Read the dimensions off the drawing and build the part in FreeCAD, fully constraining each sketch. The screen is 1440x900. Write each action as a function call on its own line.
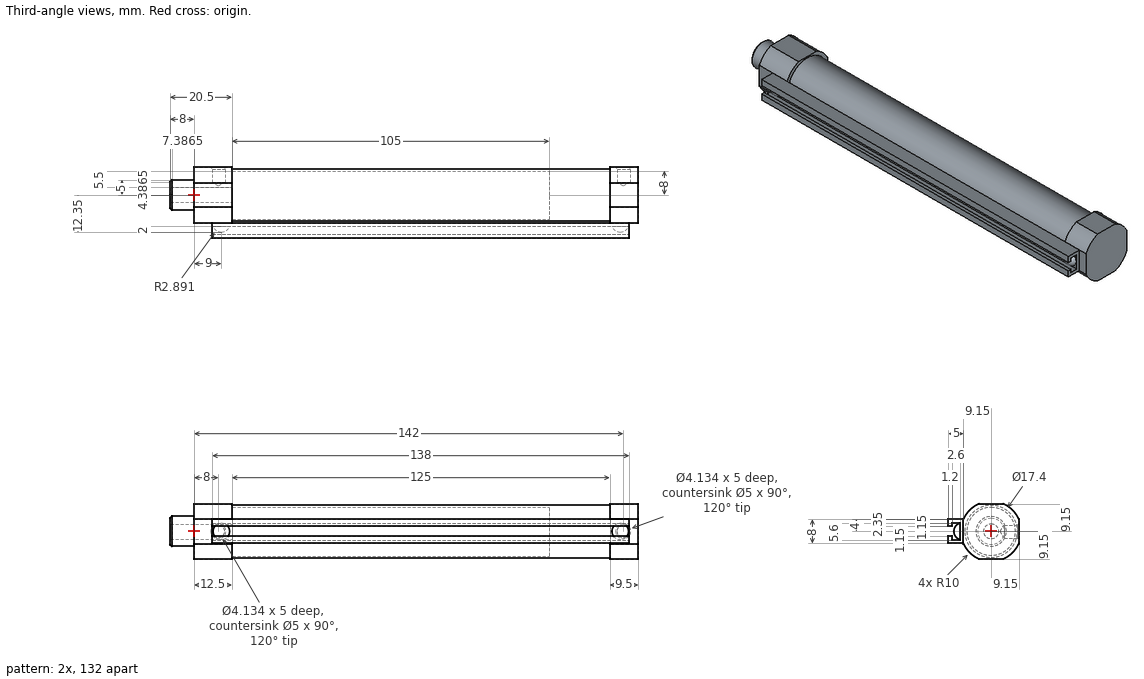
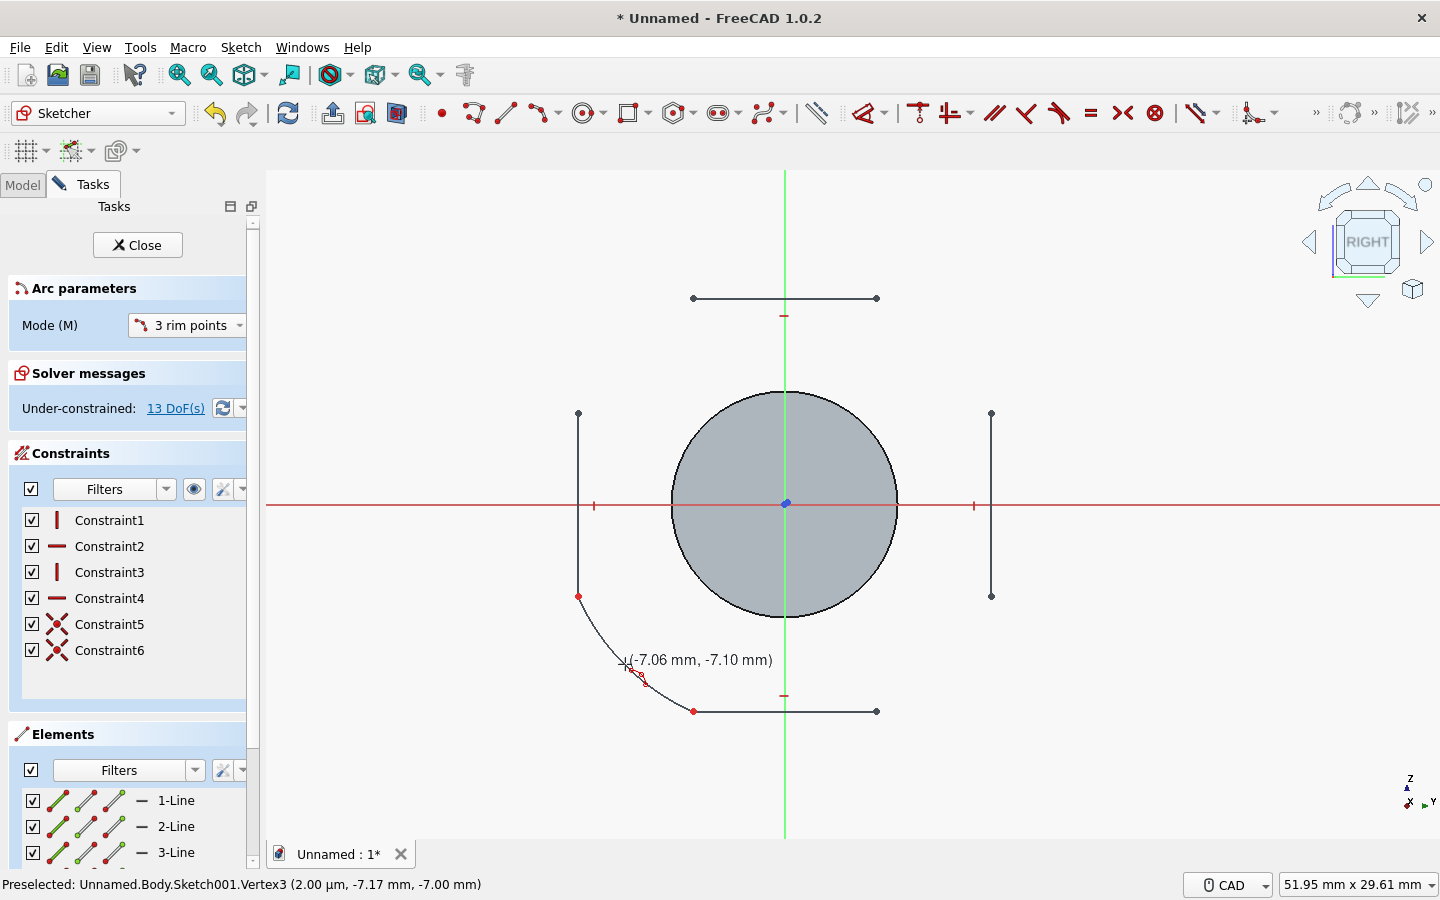
click(876, 712)
click(991, 597)
click(944, 664)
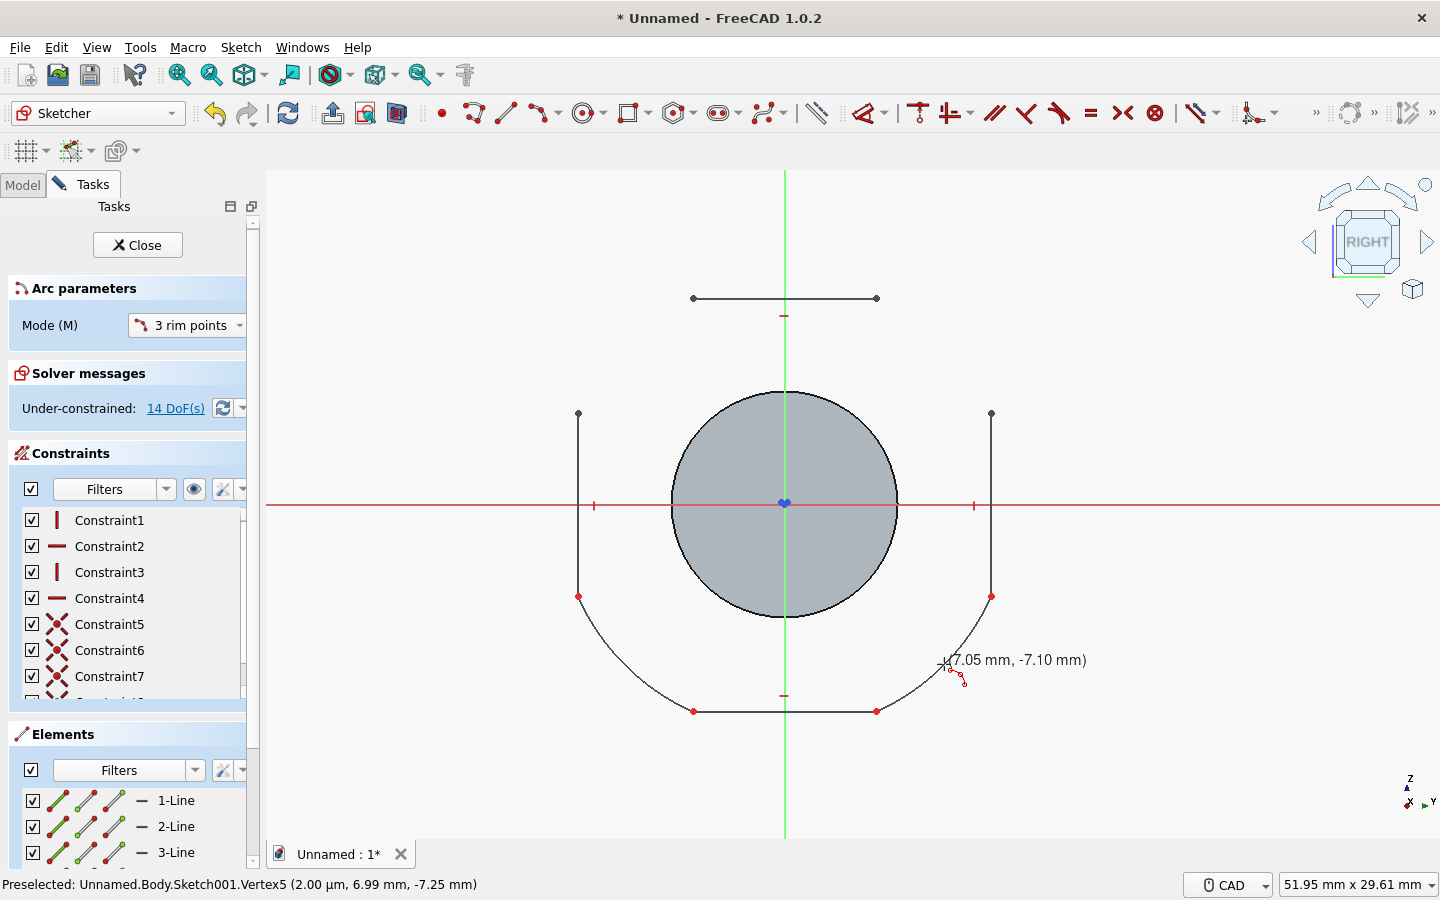
click(991, 414)
click(876, 299)
click(944, 345)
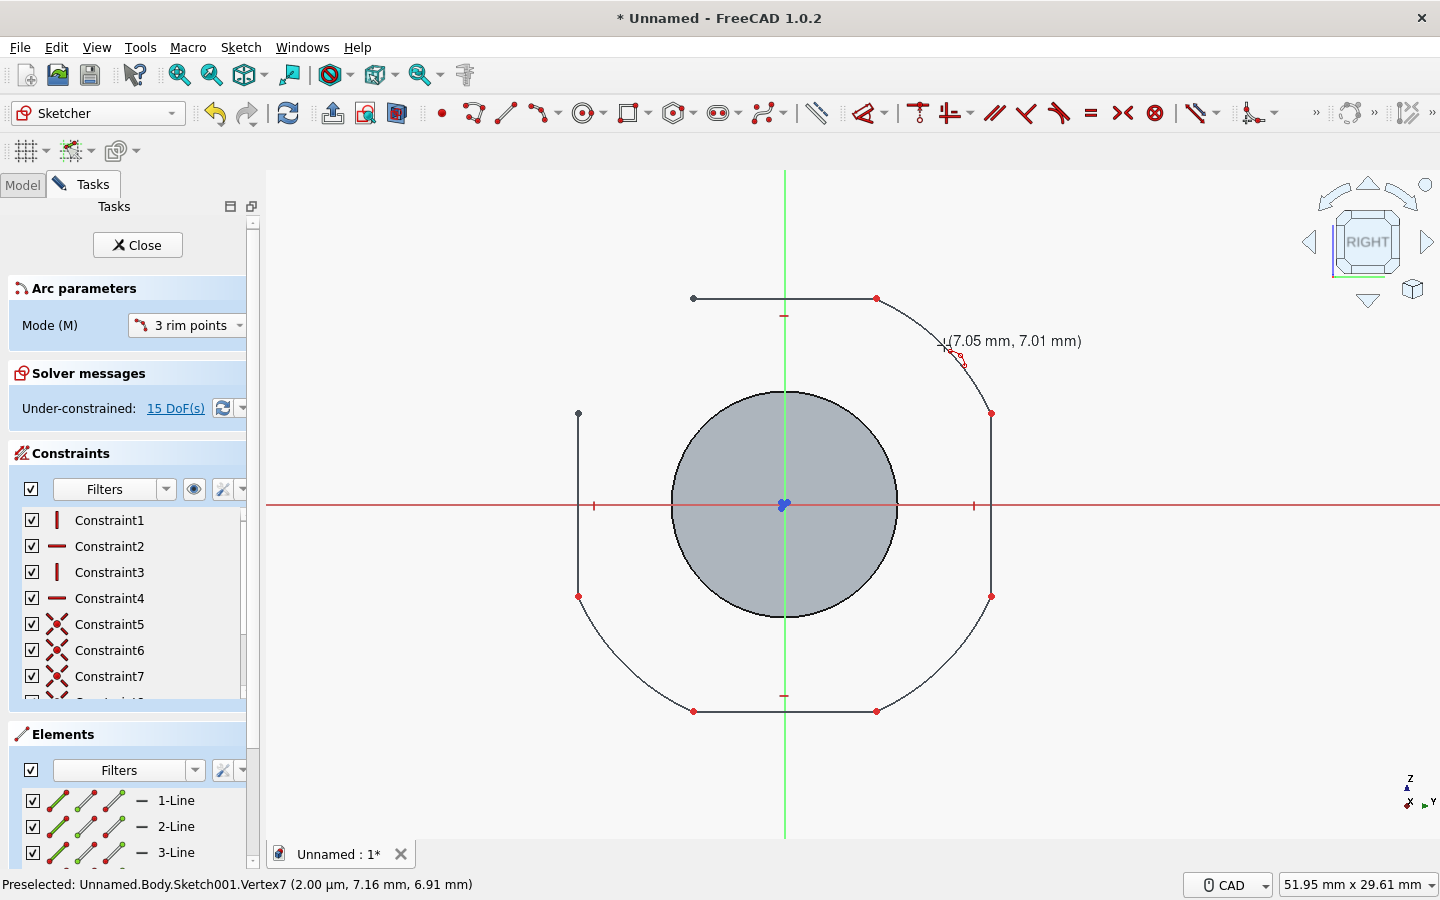
click(693, 299)
click(578, 414)
click(625, 345)
key(Escape)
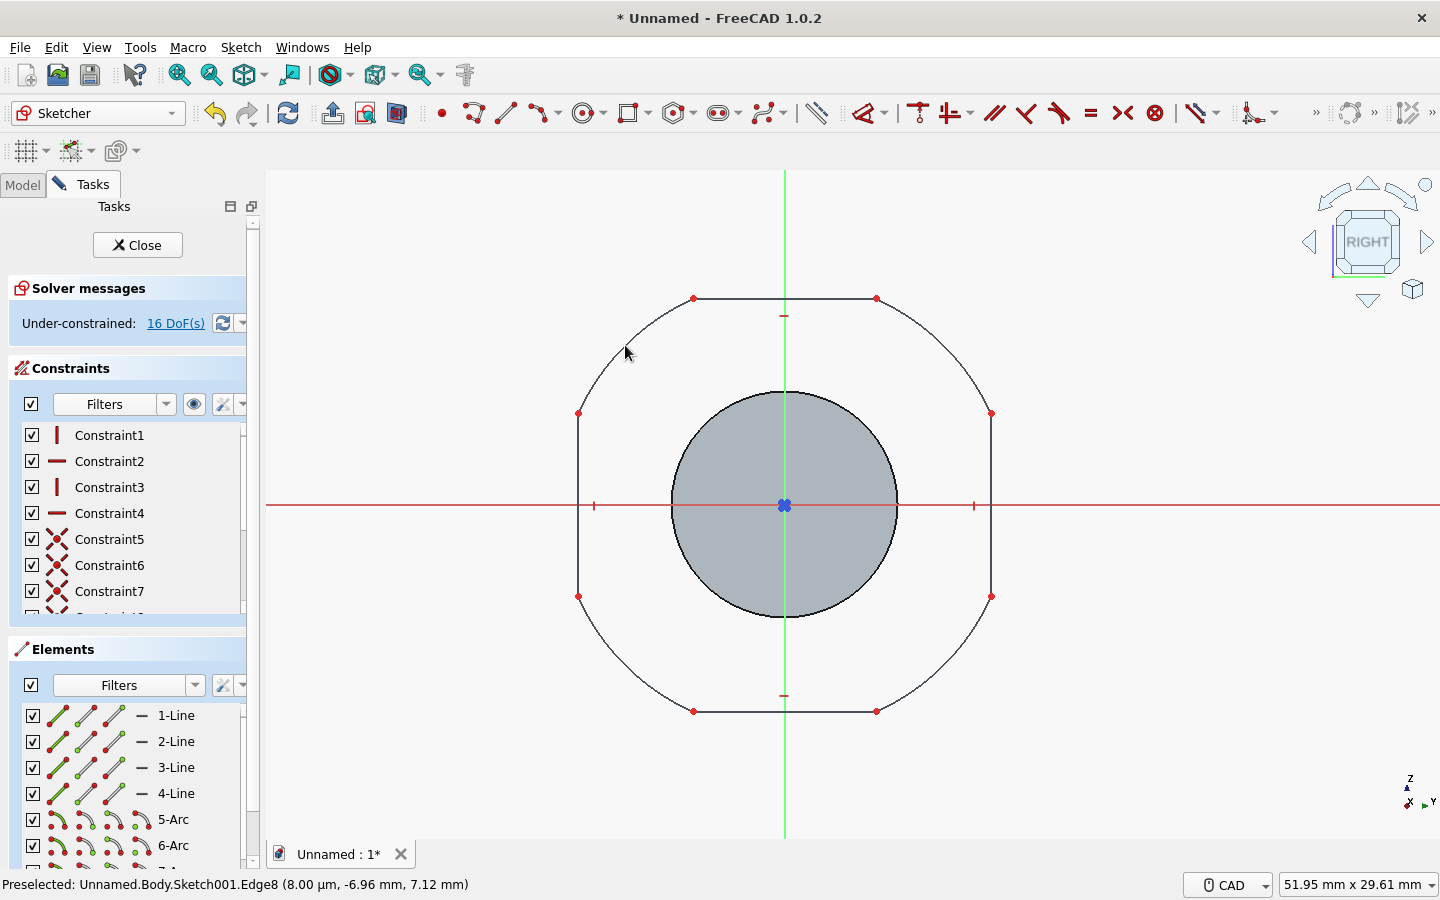
click(603, 640)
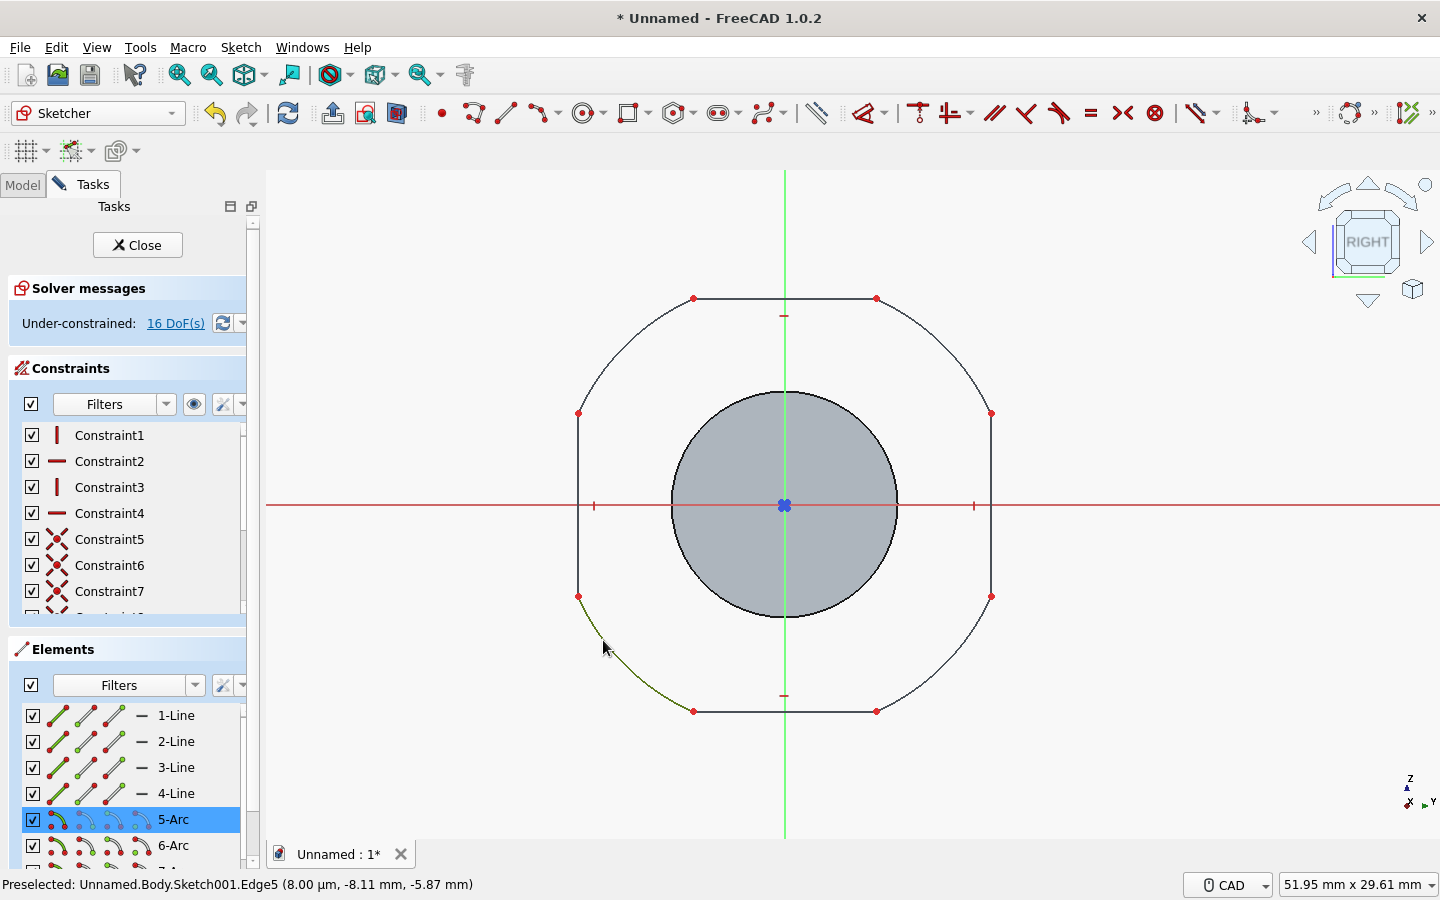
click(919, 687)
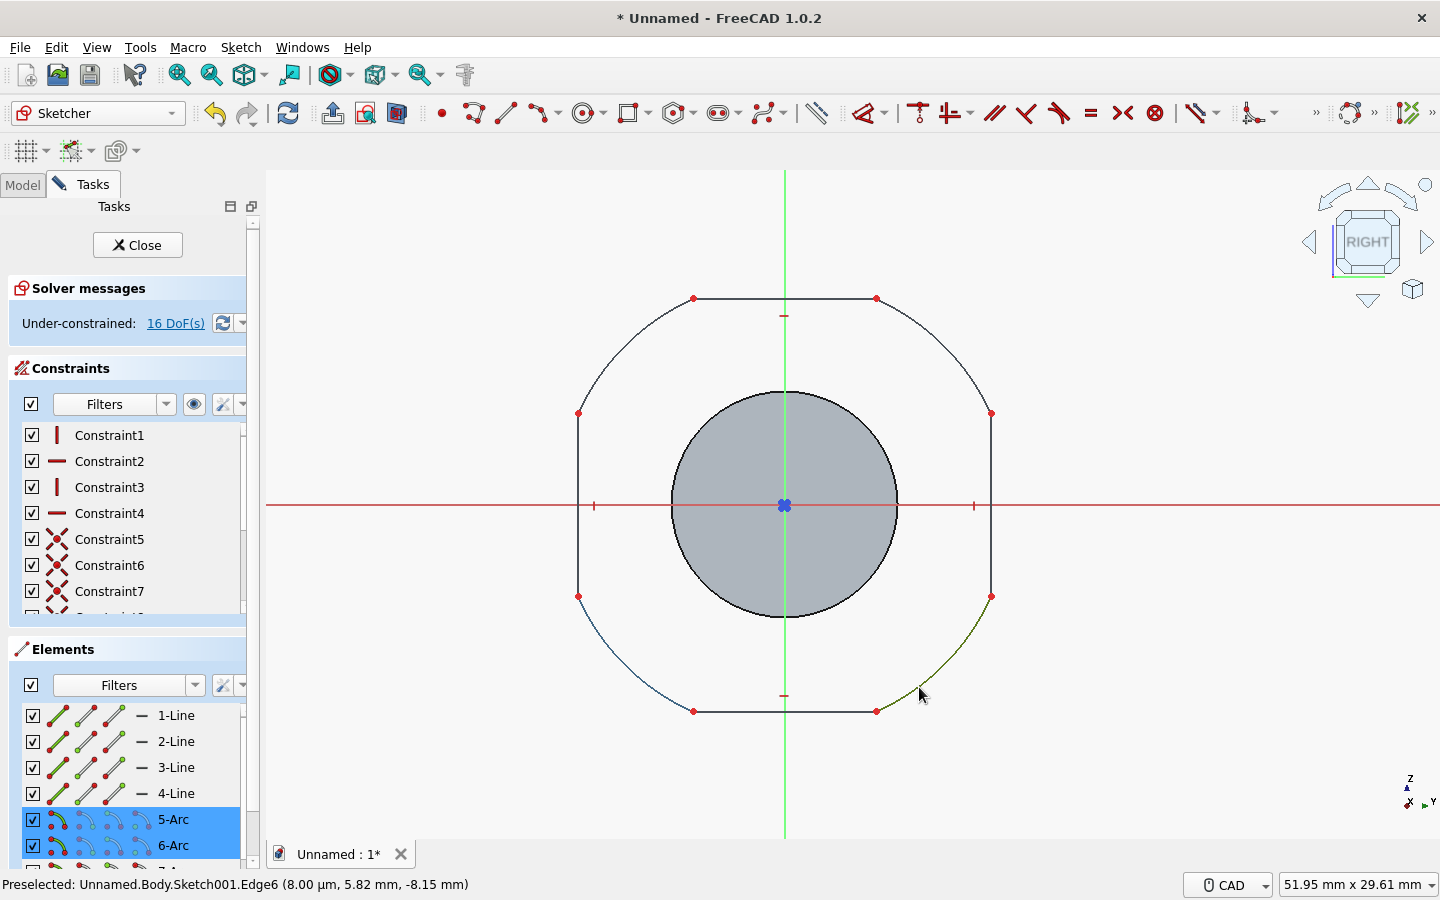
click(918, 114)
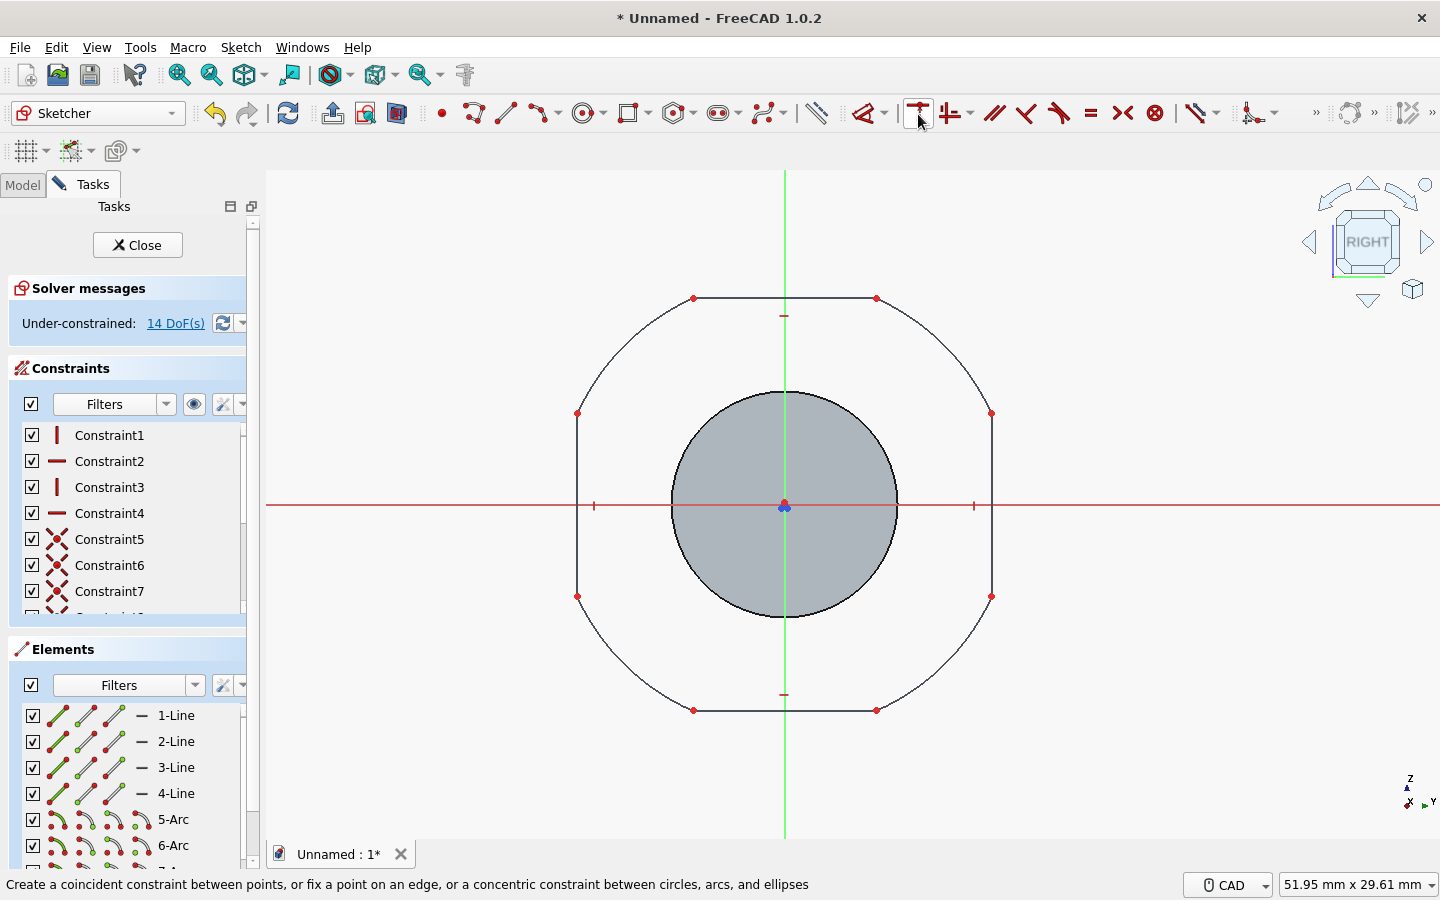
click(603, 640)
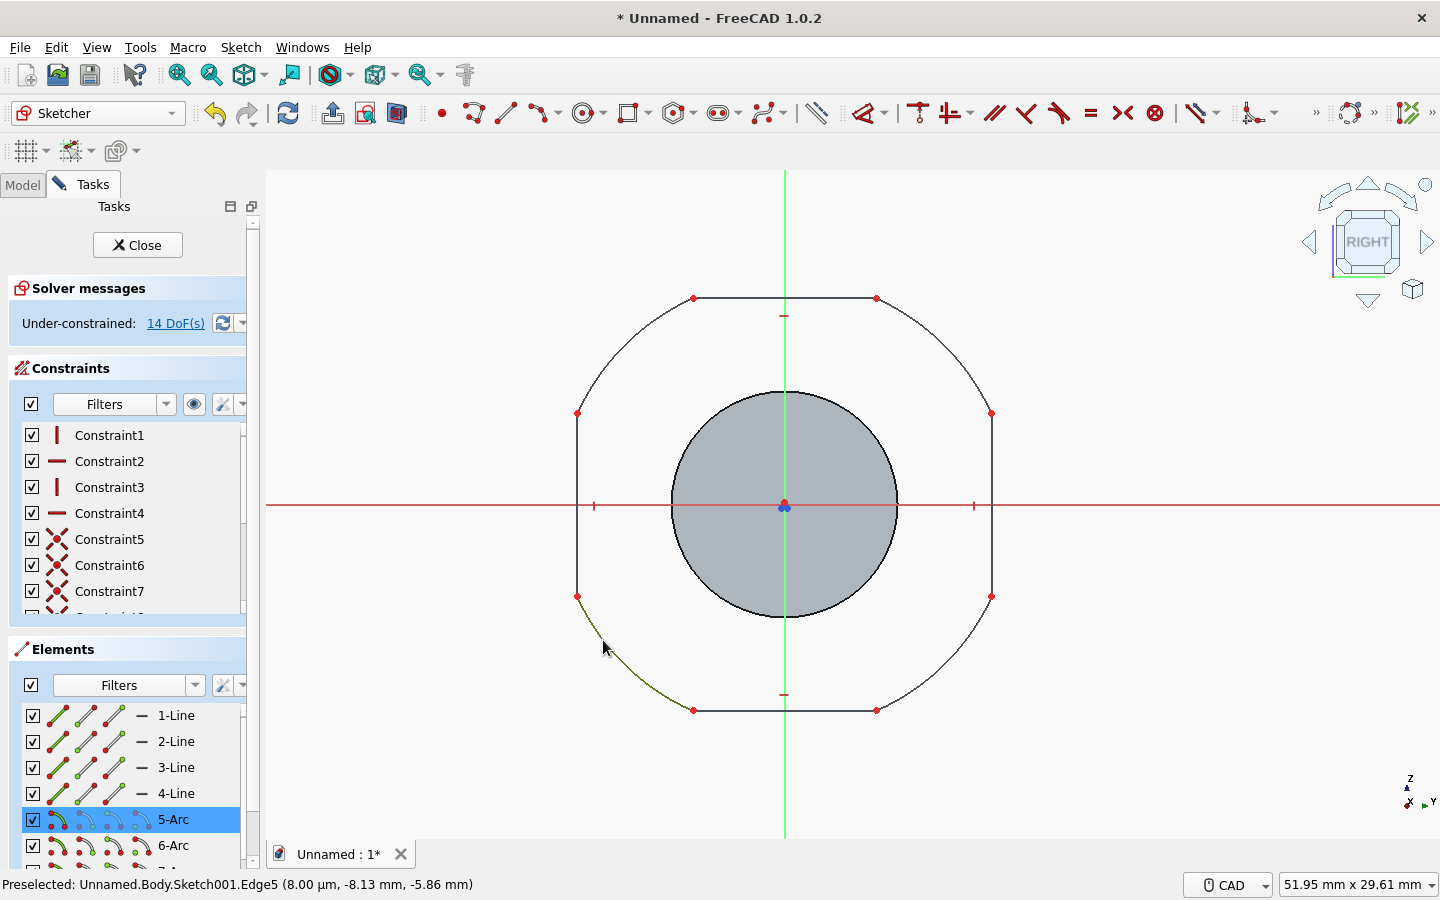
click(966, 371)